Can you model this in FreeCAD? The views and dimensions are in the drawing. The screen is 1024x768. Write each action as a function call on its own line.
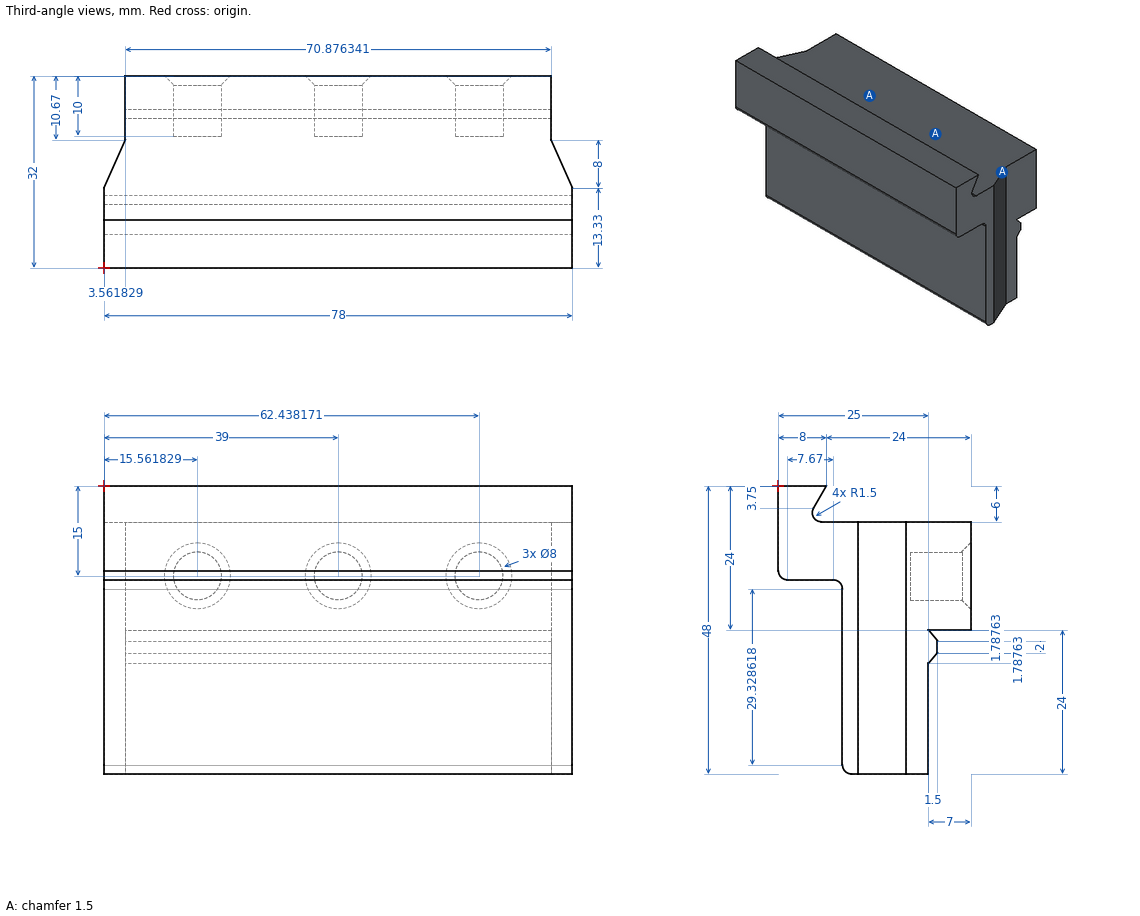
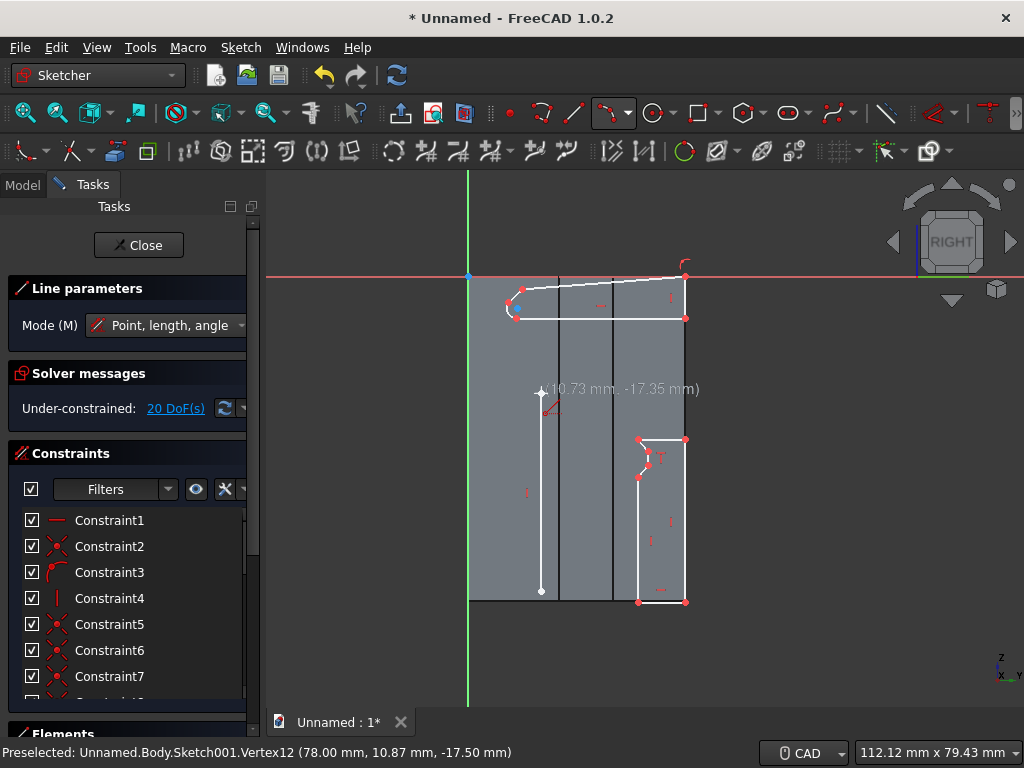
click(530, 383)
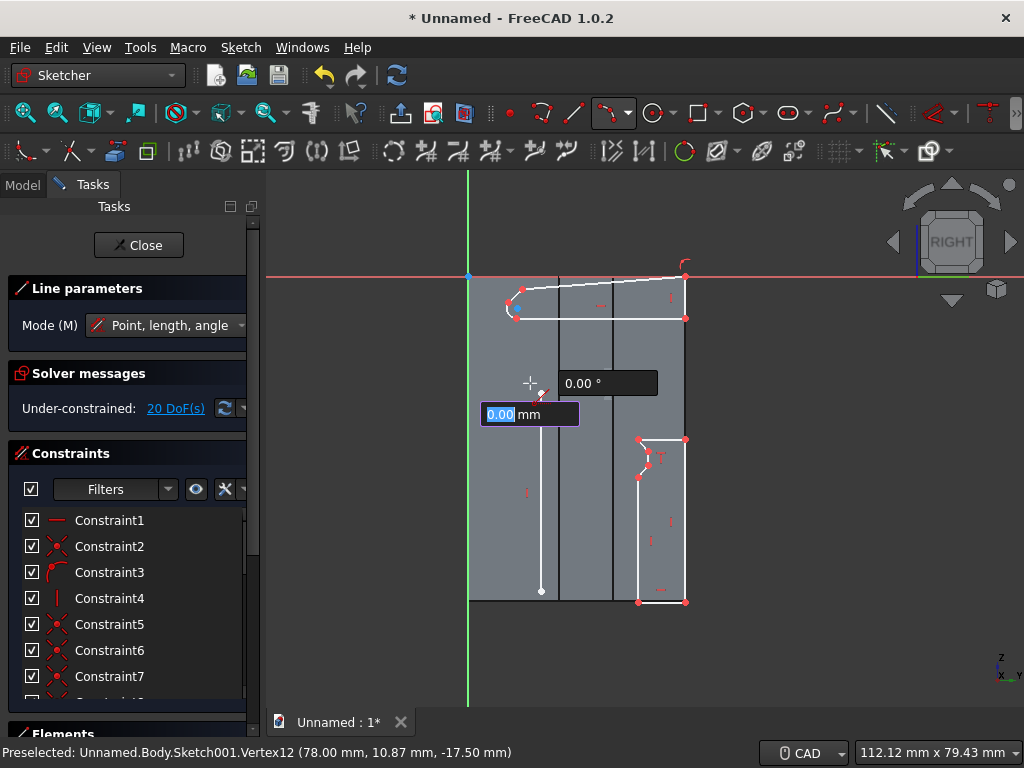
scroll(479, 383, up, 3)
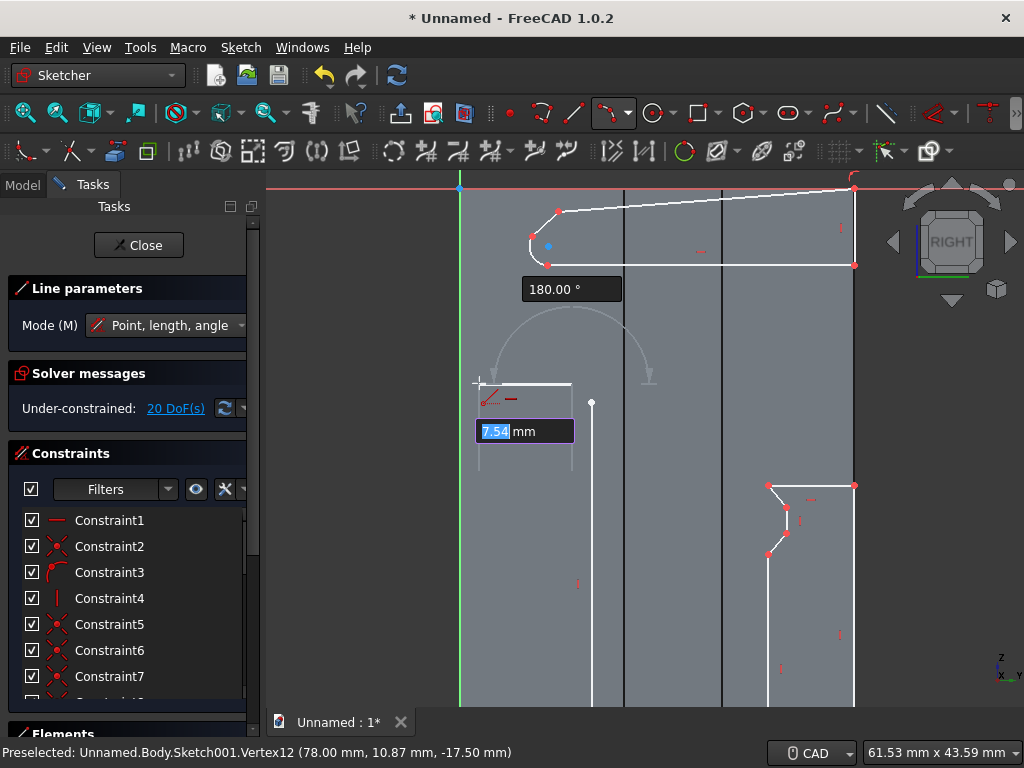
click(478, 383)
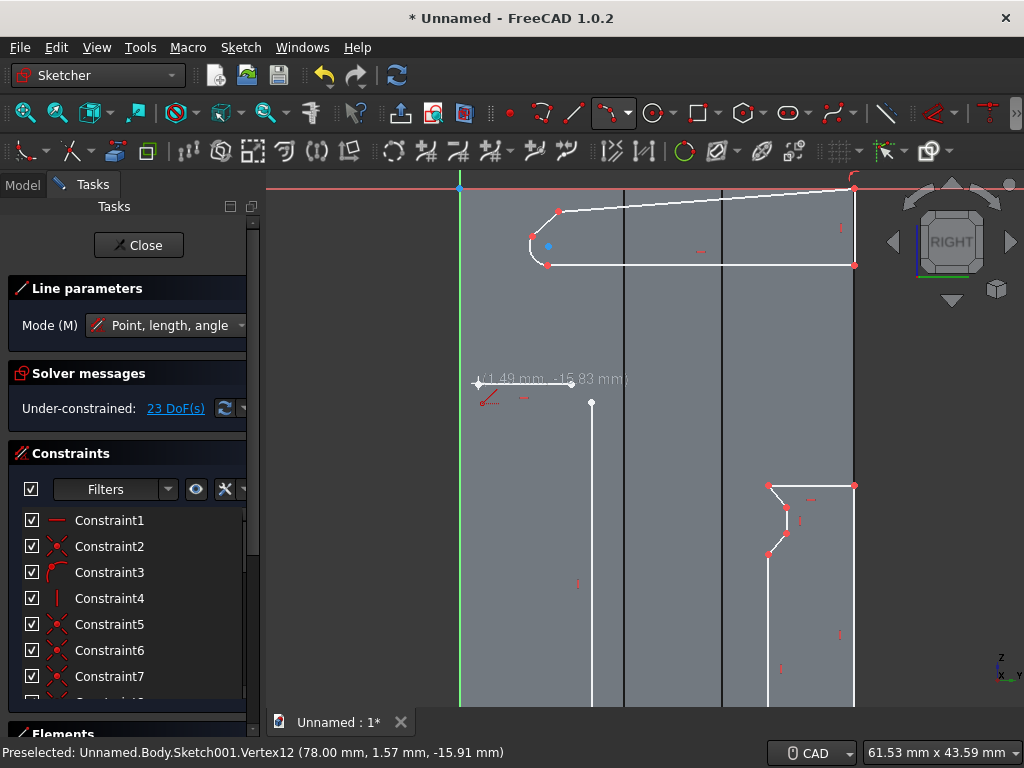
click(542, 114)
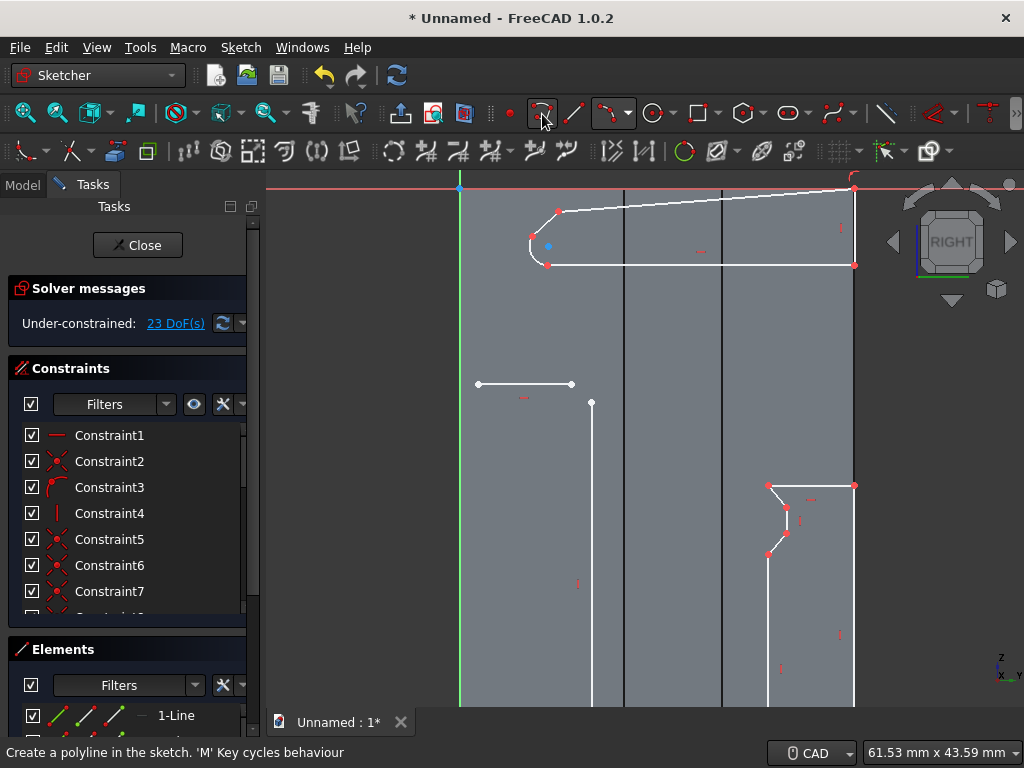
click(460, 364)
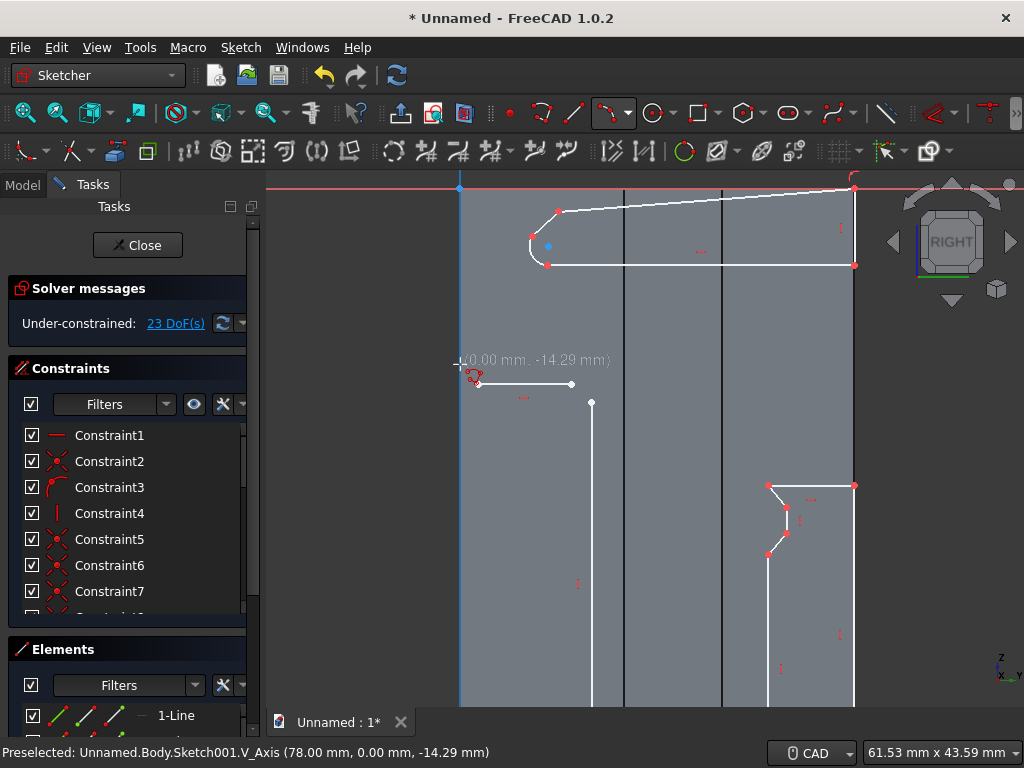
scroll(479, 382, down, 3)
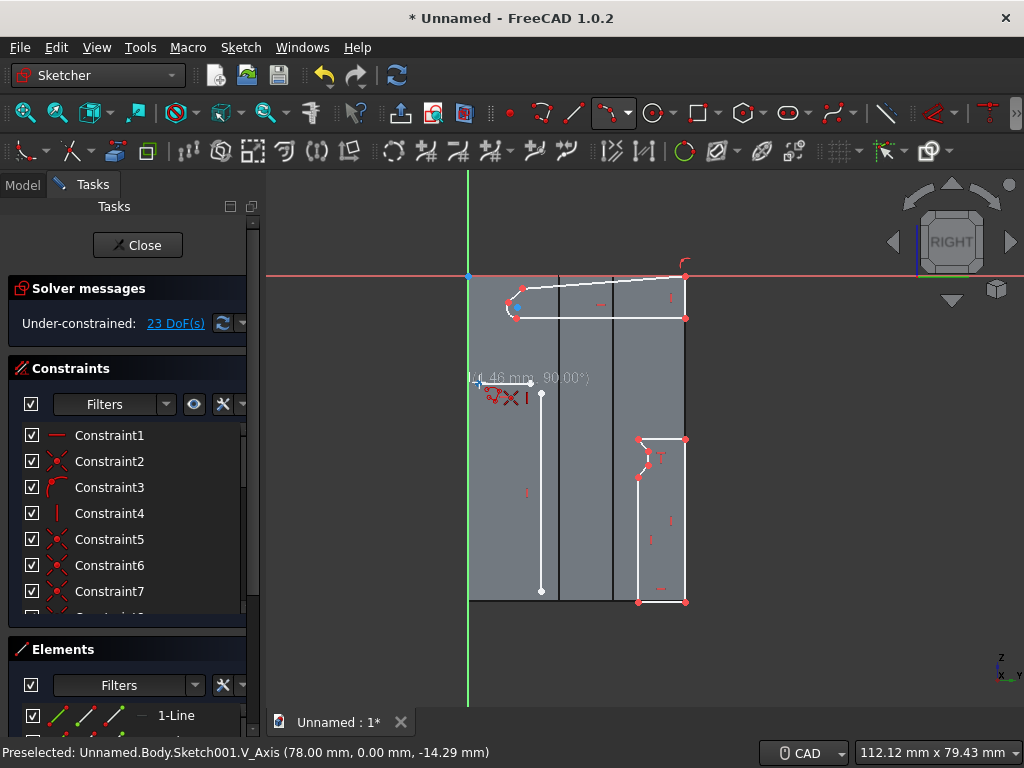
click(477, 601)
click(551, 601)
right_click(551, 601)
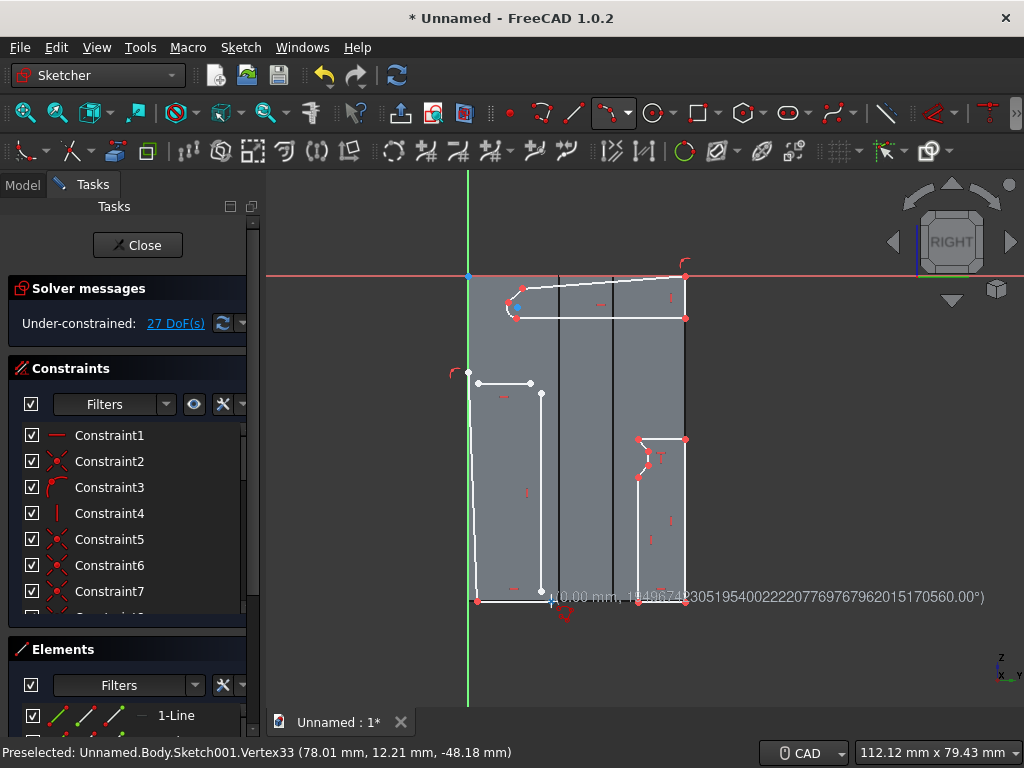
click(608, 114)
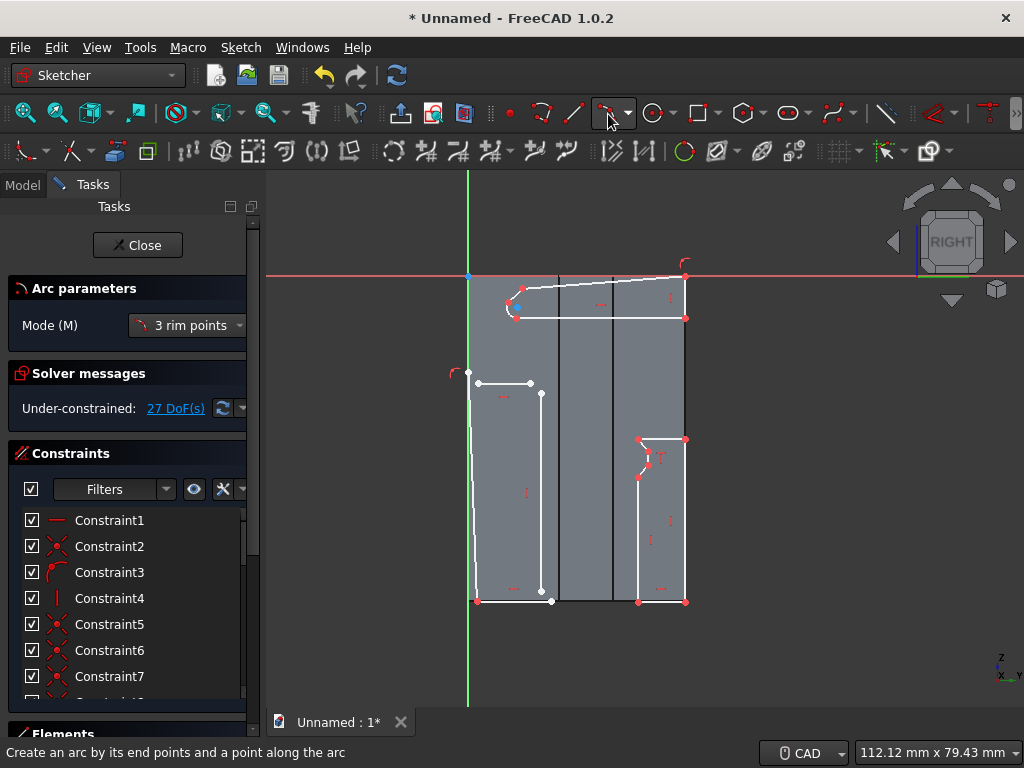
click(541, 394)
click(530, 384)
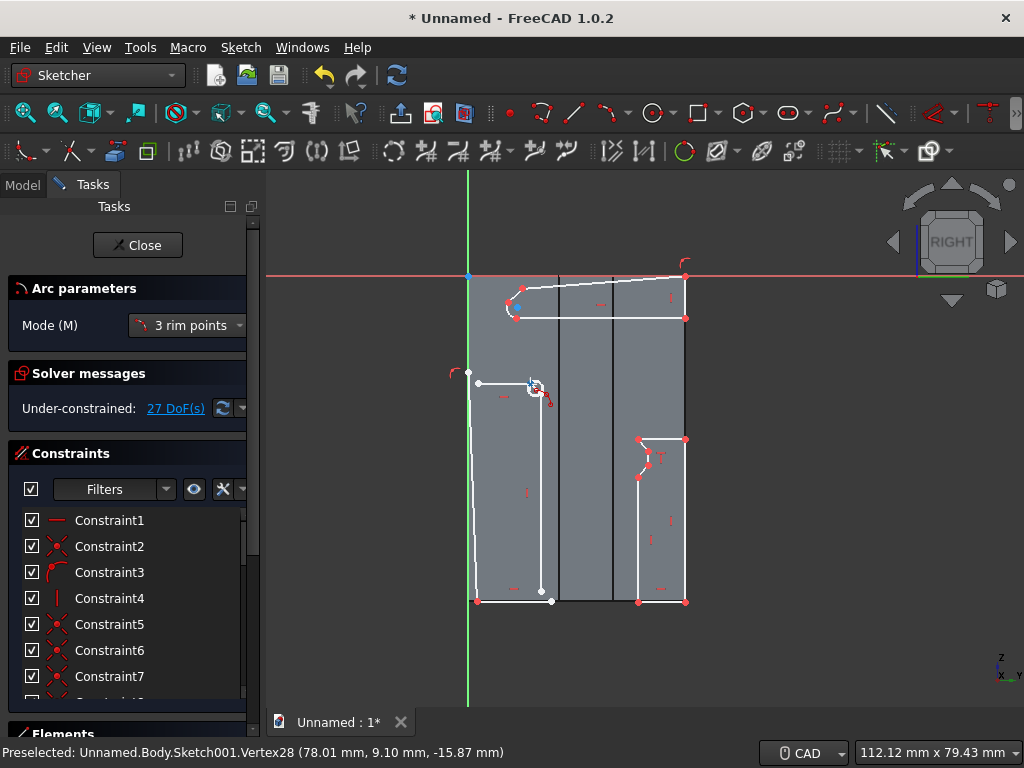
scroll(538, 385, up, 9)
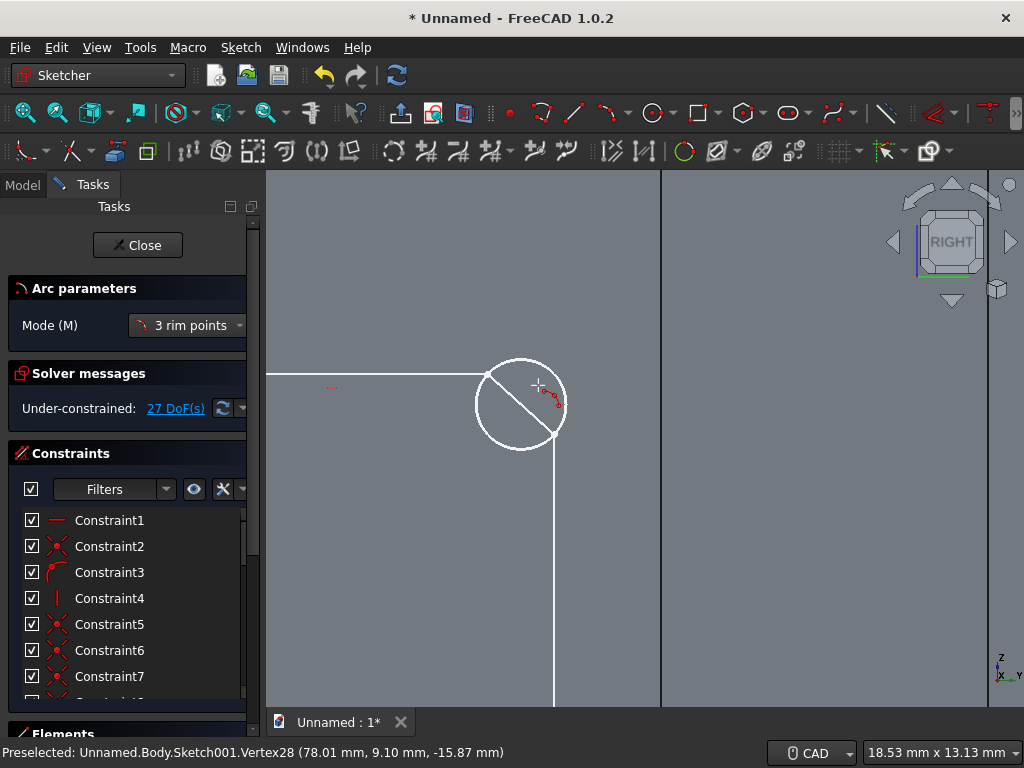
click(534, 384)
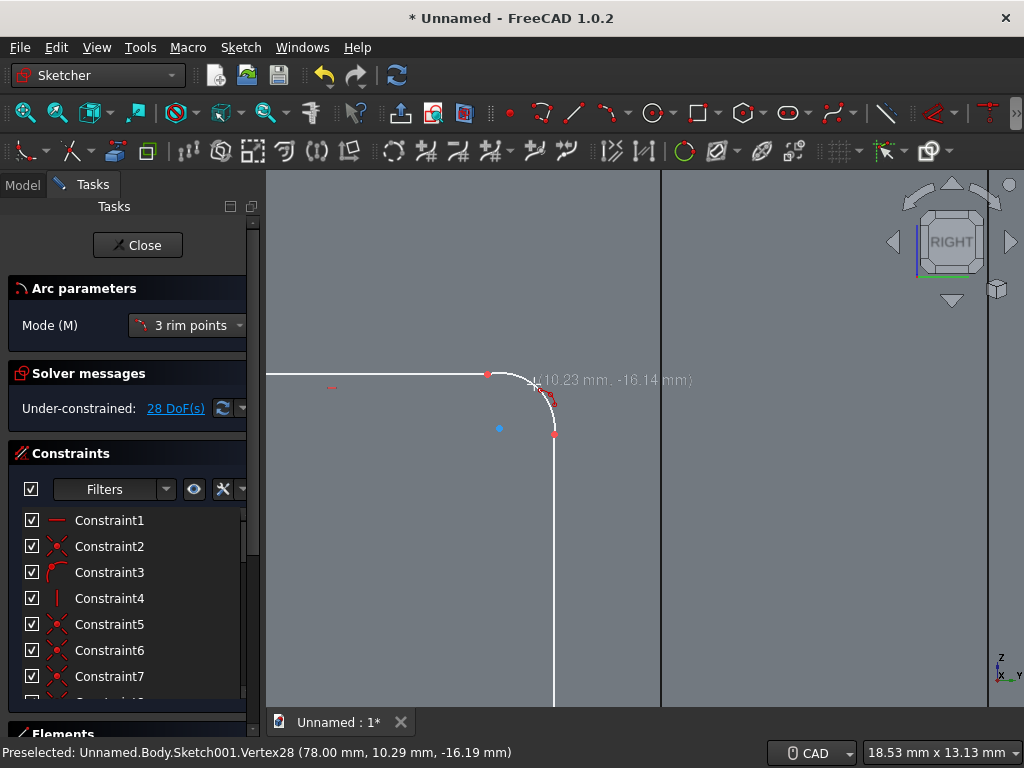
scroll(538, 385, down, 9)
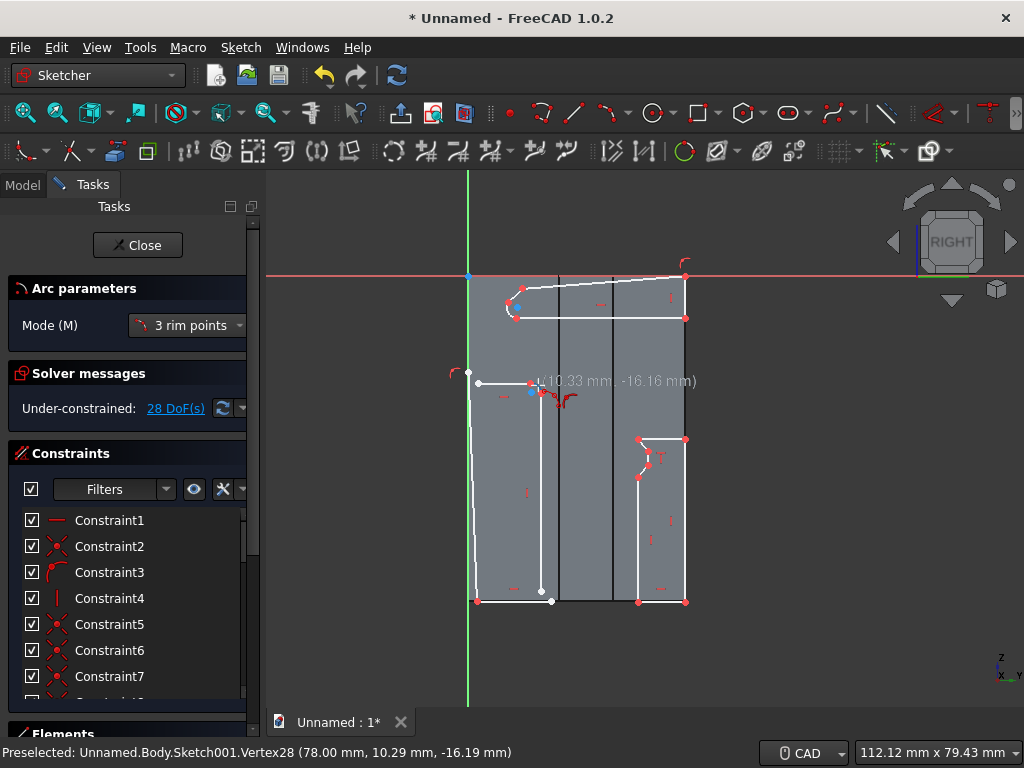
scroll(479, 382, up, 3)